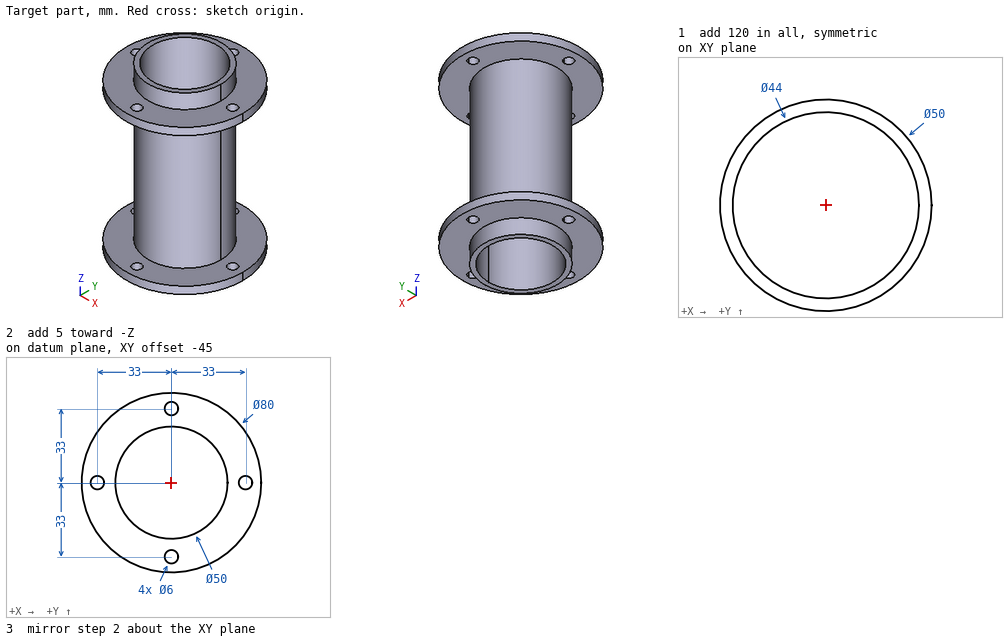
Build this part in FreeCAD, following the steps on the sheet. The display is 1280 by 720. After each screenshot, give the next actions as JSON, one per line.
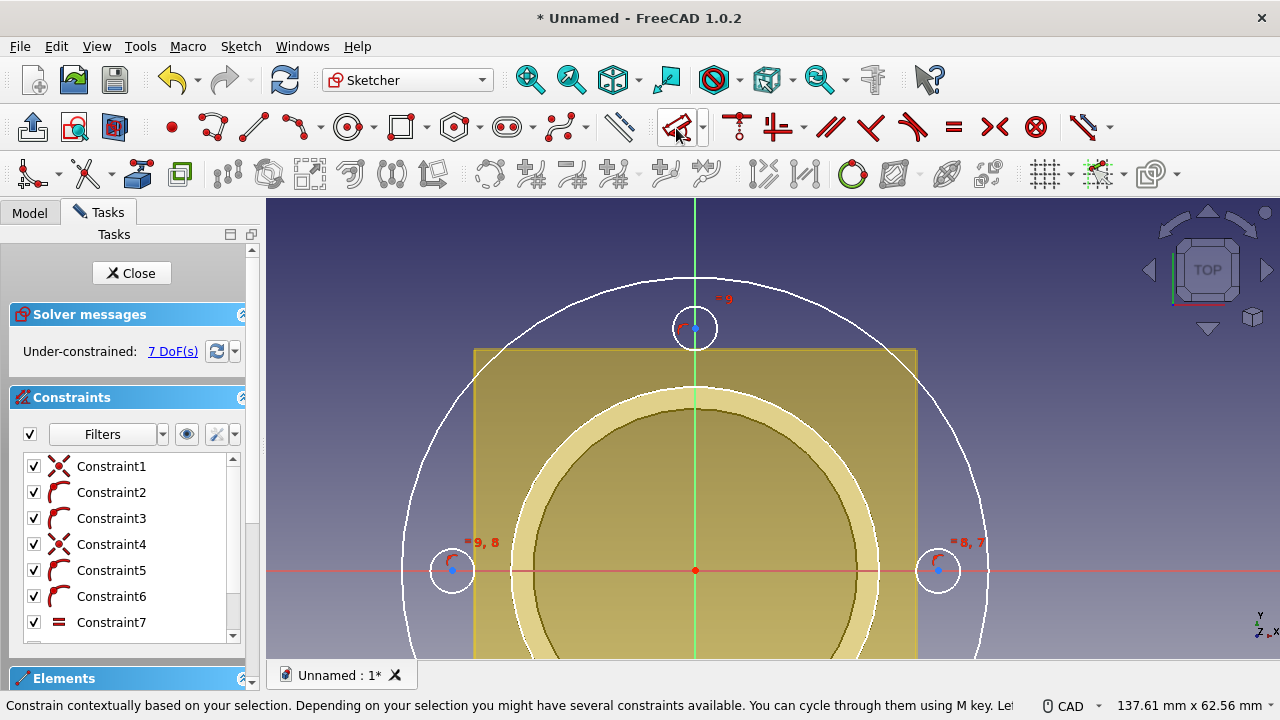
{"action": "left_click", "coordinate": [902, 363]}
{"action": "left_click", "coordinate": [925, 340]}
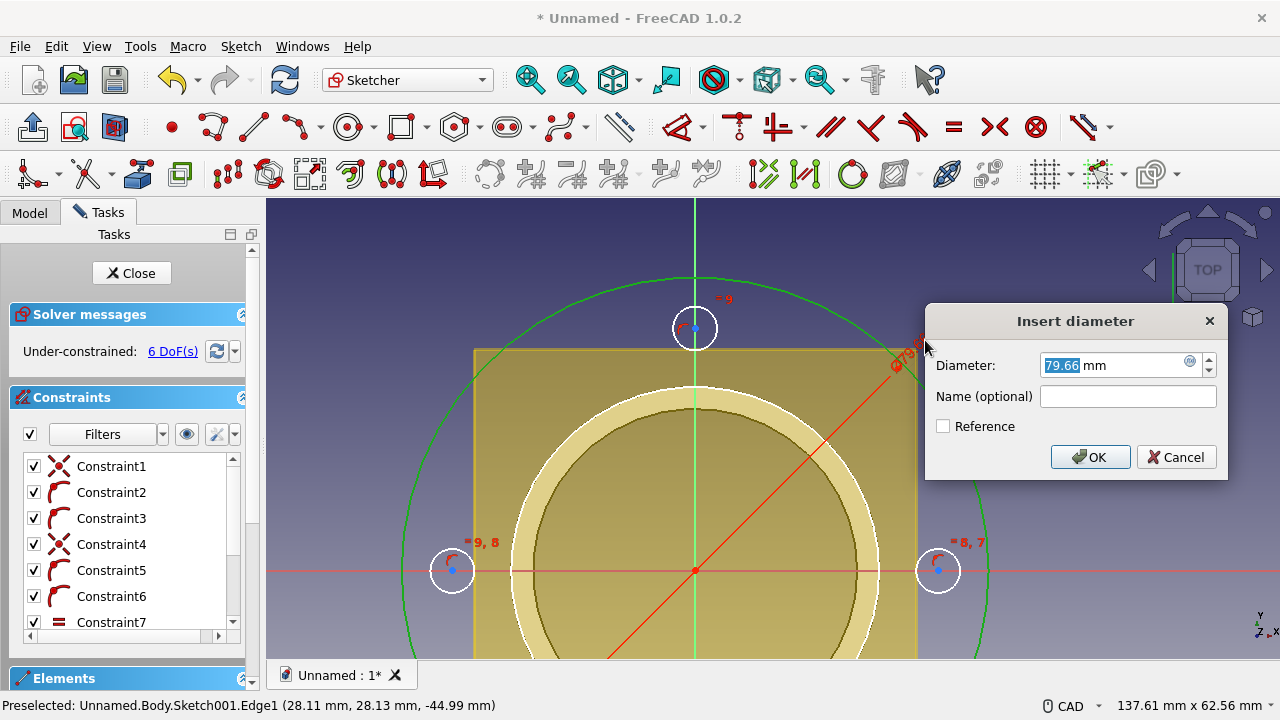
{"action": "type", "text": "80"}
{"action": "key", "text": "Return"}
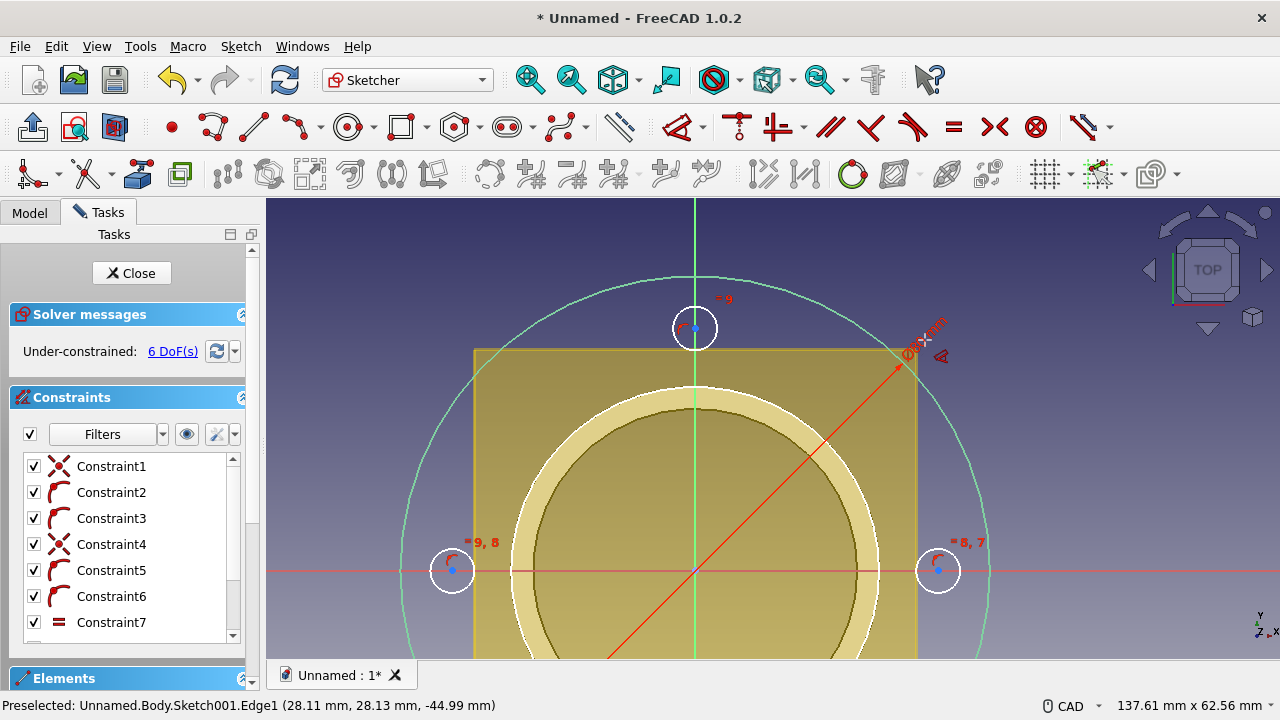
{"action": "scroll", "coordinate": [712, 312], "scroll_direction": "down", "scroll_amount": 4}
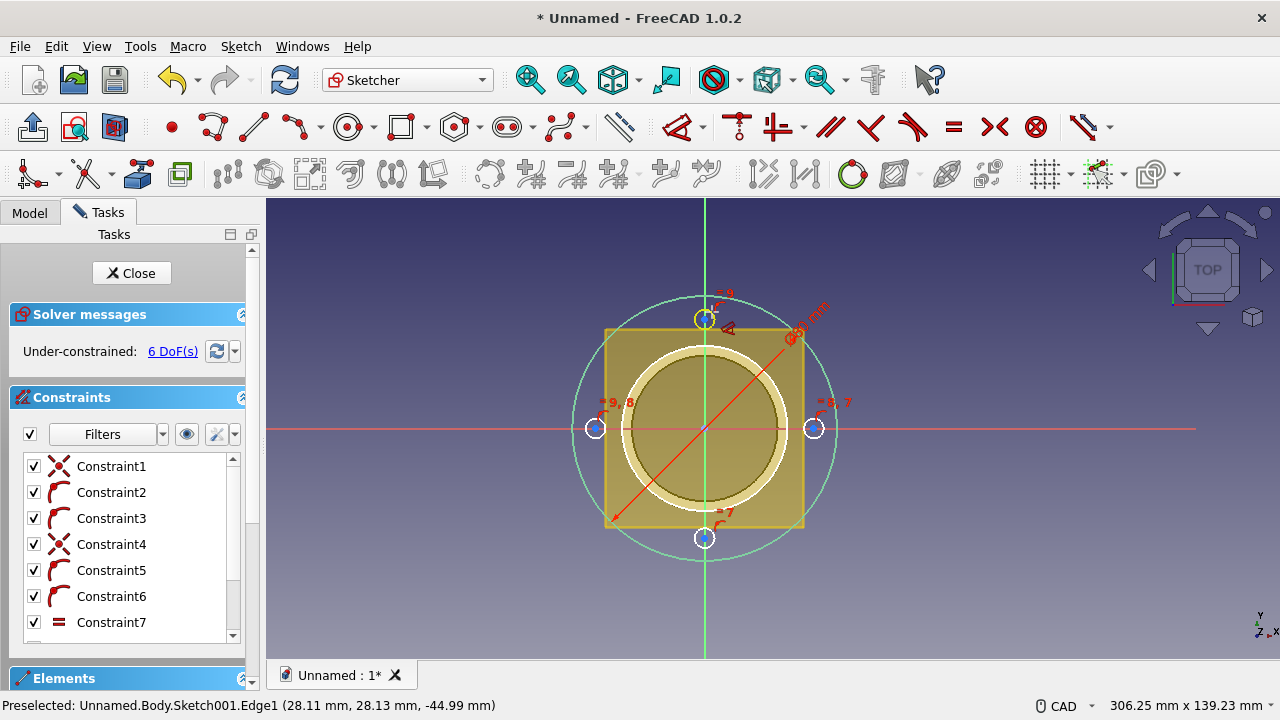
{"action": "scroll", "coordinate": [712, 531], "scroll_direction": "up", "scroll_amount": 4}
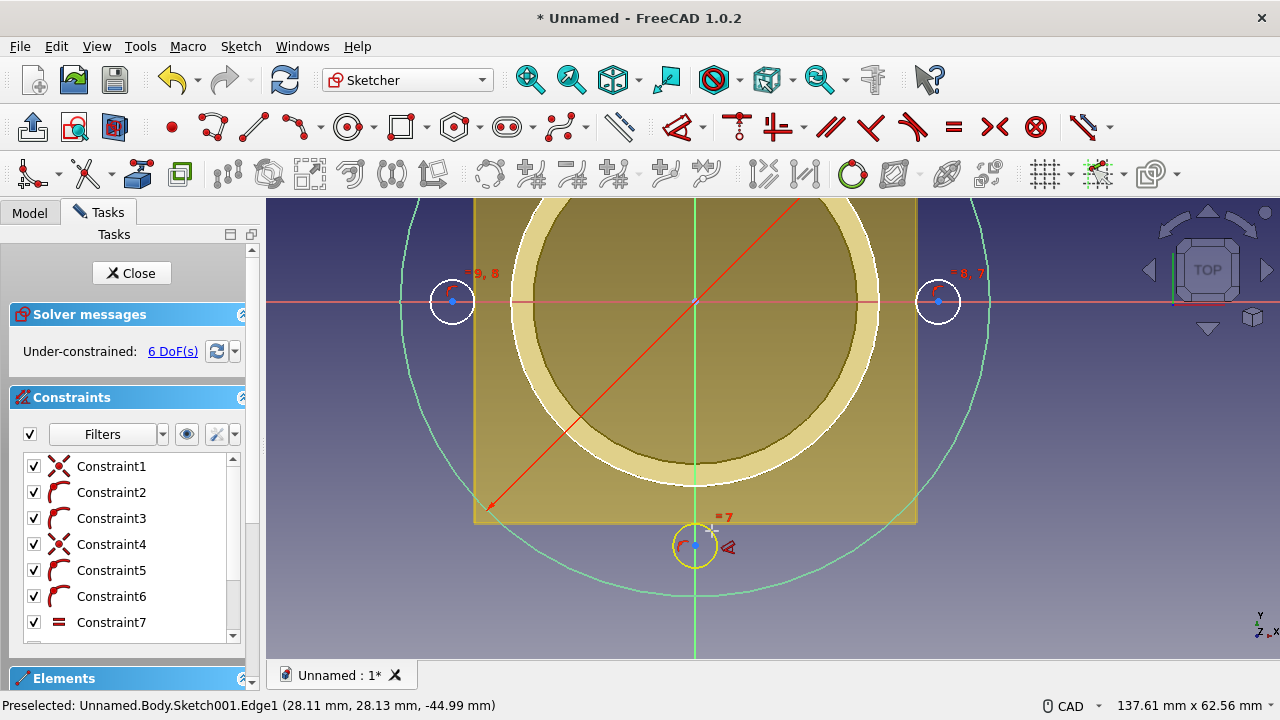
{"action": "left_click", "coordinate": [711, 530]}
{"action": "left_click", "coordinate": [734, 507]}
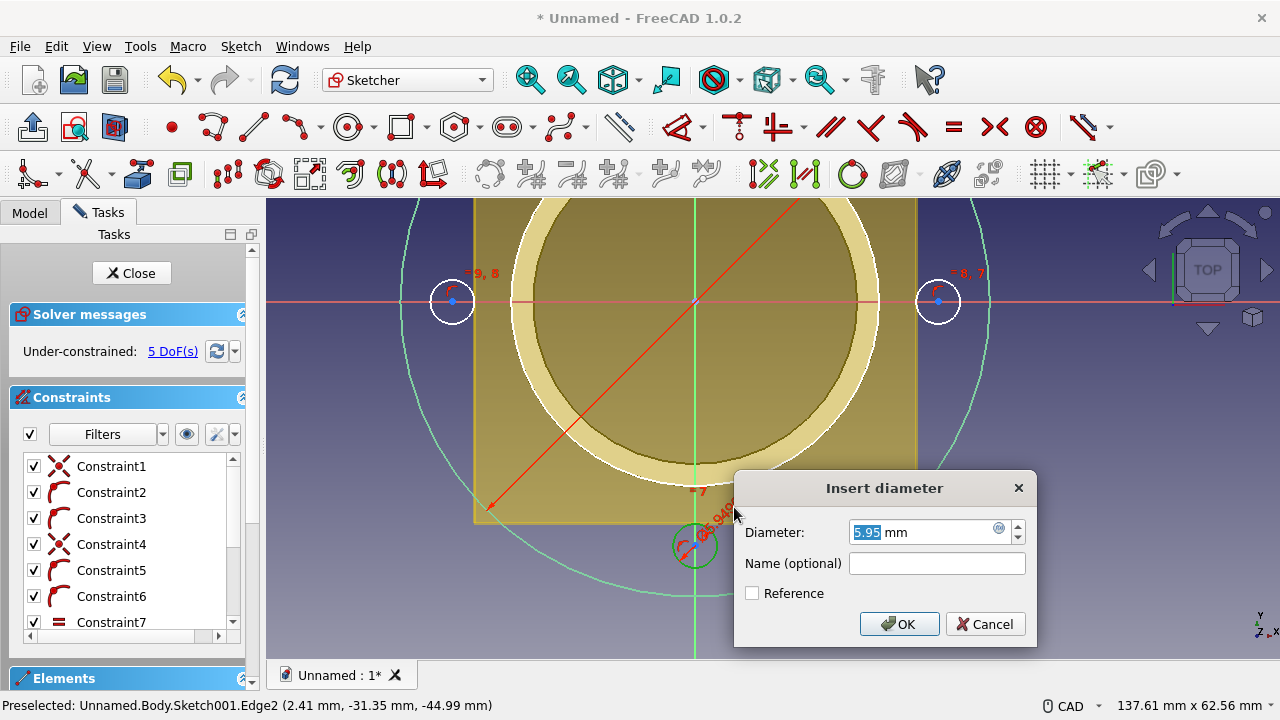
{"action": "type", "text": "6"}
{"action": "key", "text": "Return"}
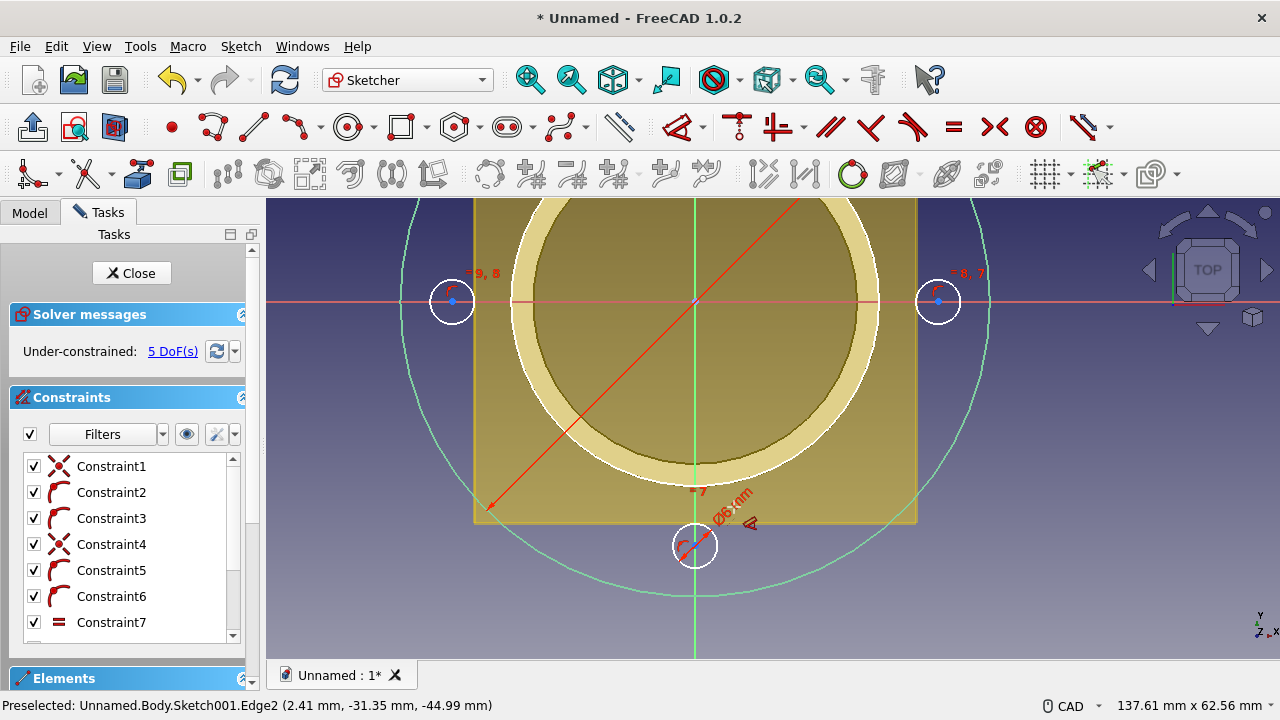
{"action": "left_click", "coordinate": [565, 432]}
{"action": "left_click", "coordinate": [542, 455]}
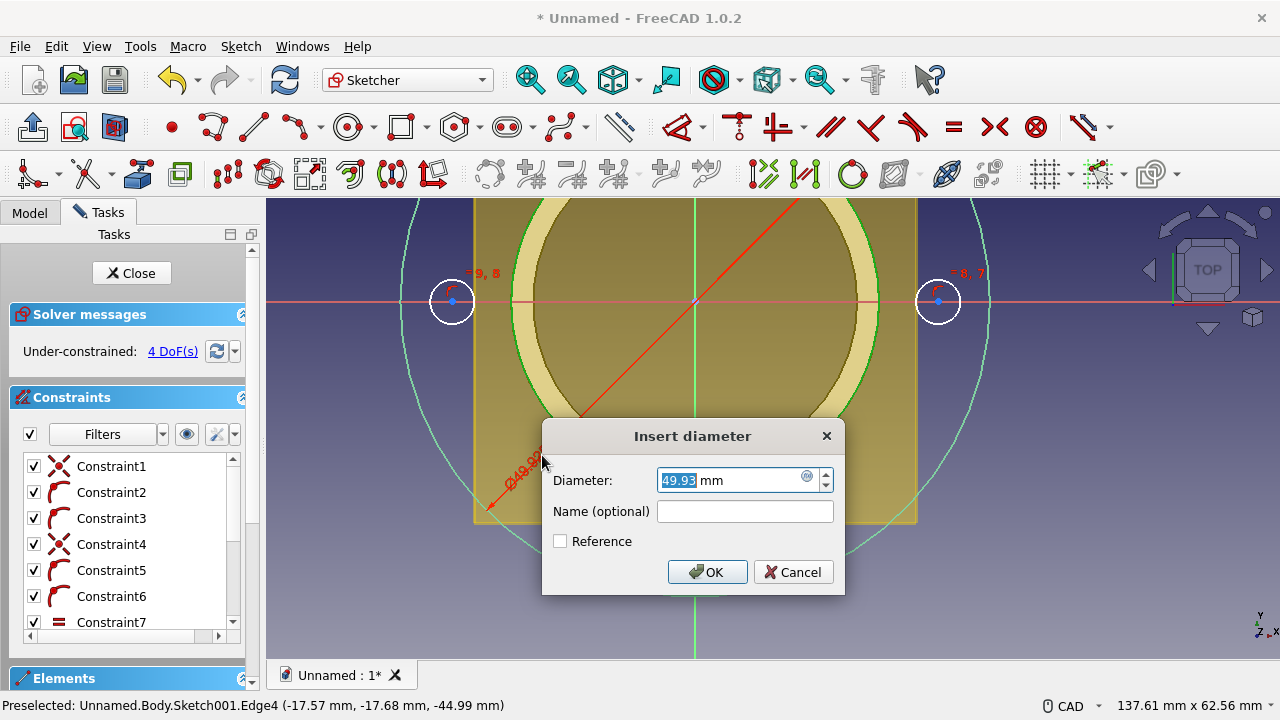
{"action": "type", "text": "50"}
{"action": "key", "text": "Return"}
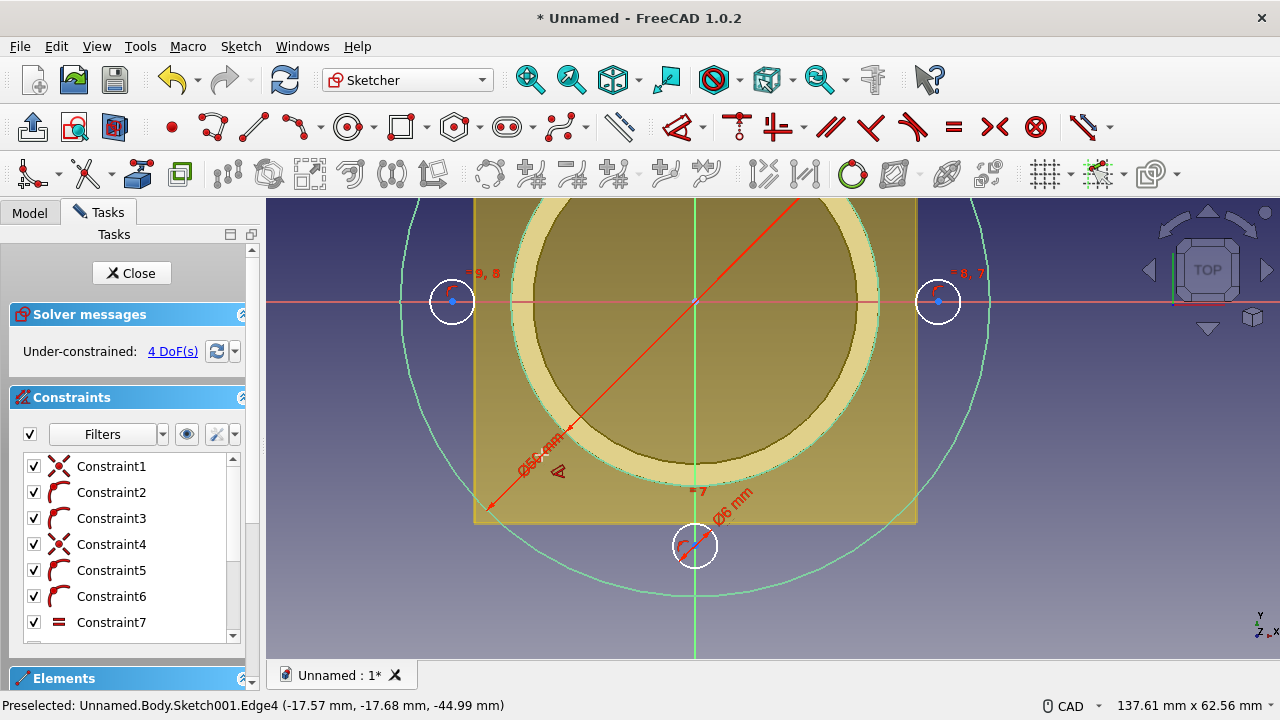
{"action": "left_click", "coordinate": [695, 546]}
{"action": "left_click", "coordinate": [729, 424]}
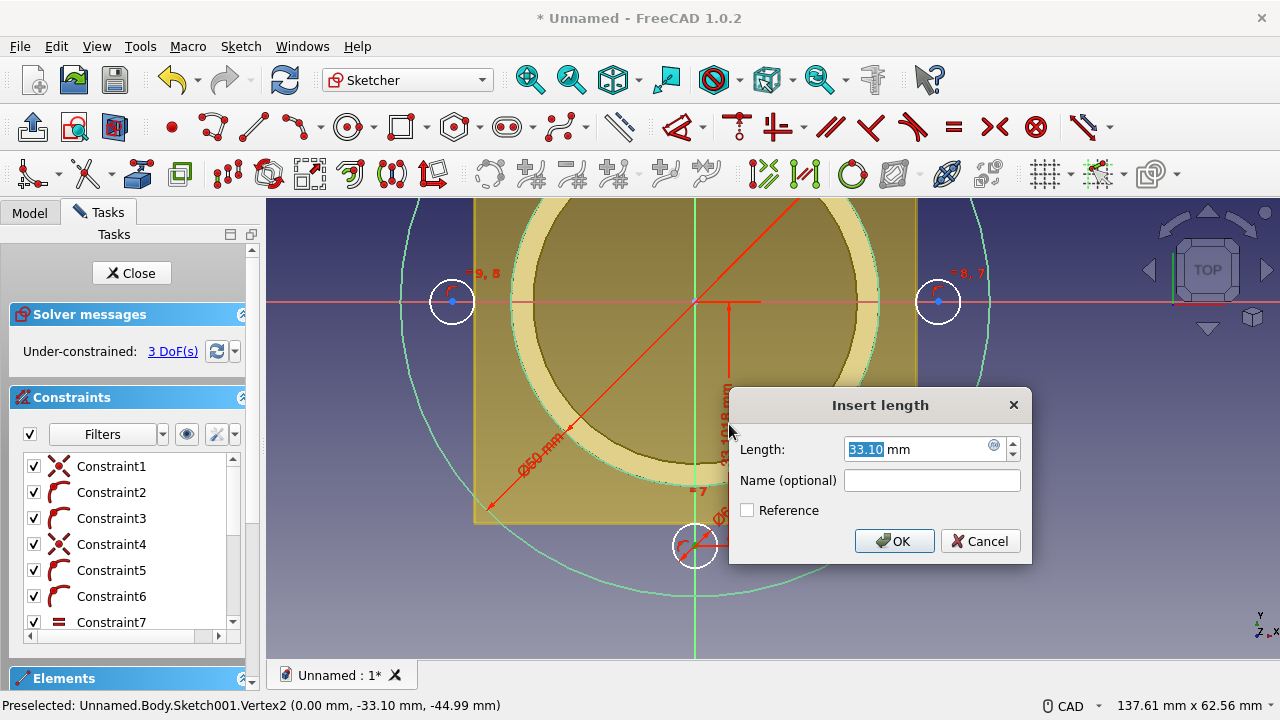
{"action": "type", "text": "33"}
{"action": "key", "text": "Return"}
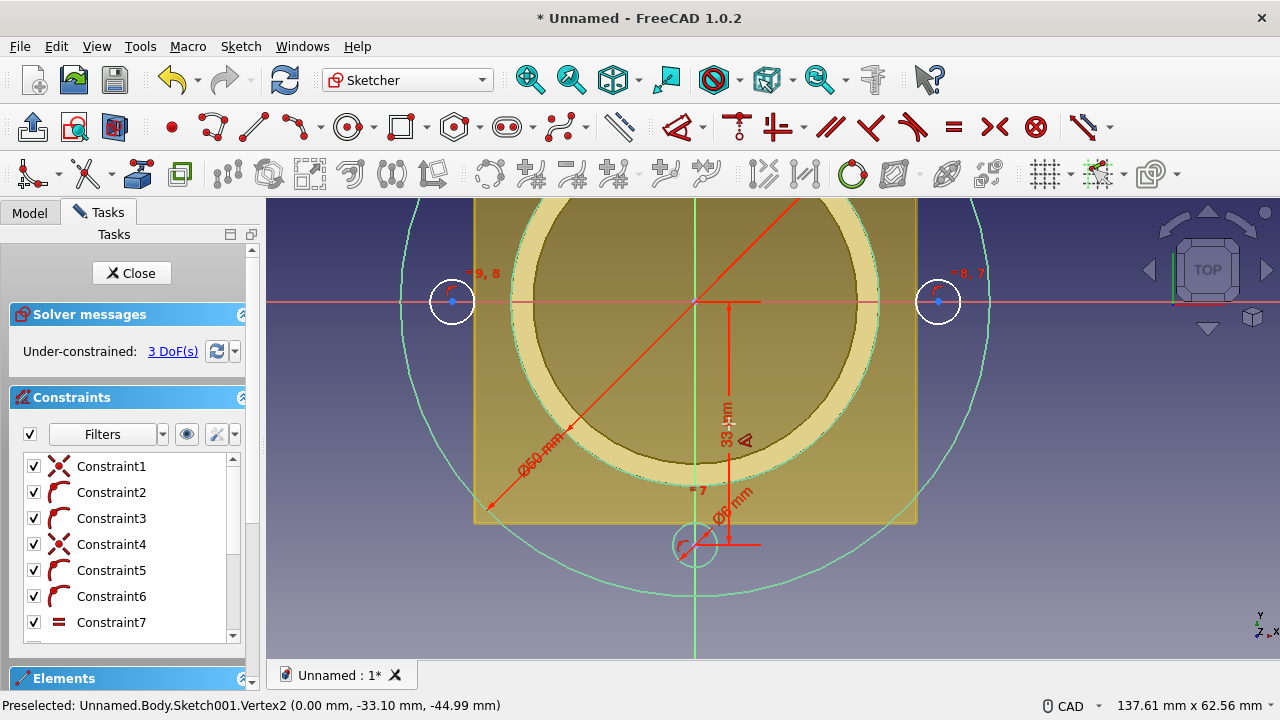
{"action": "left_click", "coordinate": [938, 302]}
{"action": "left_click", "coordinate": [817, 336]}